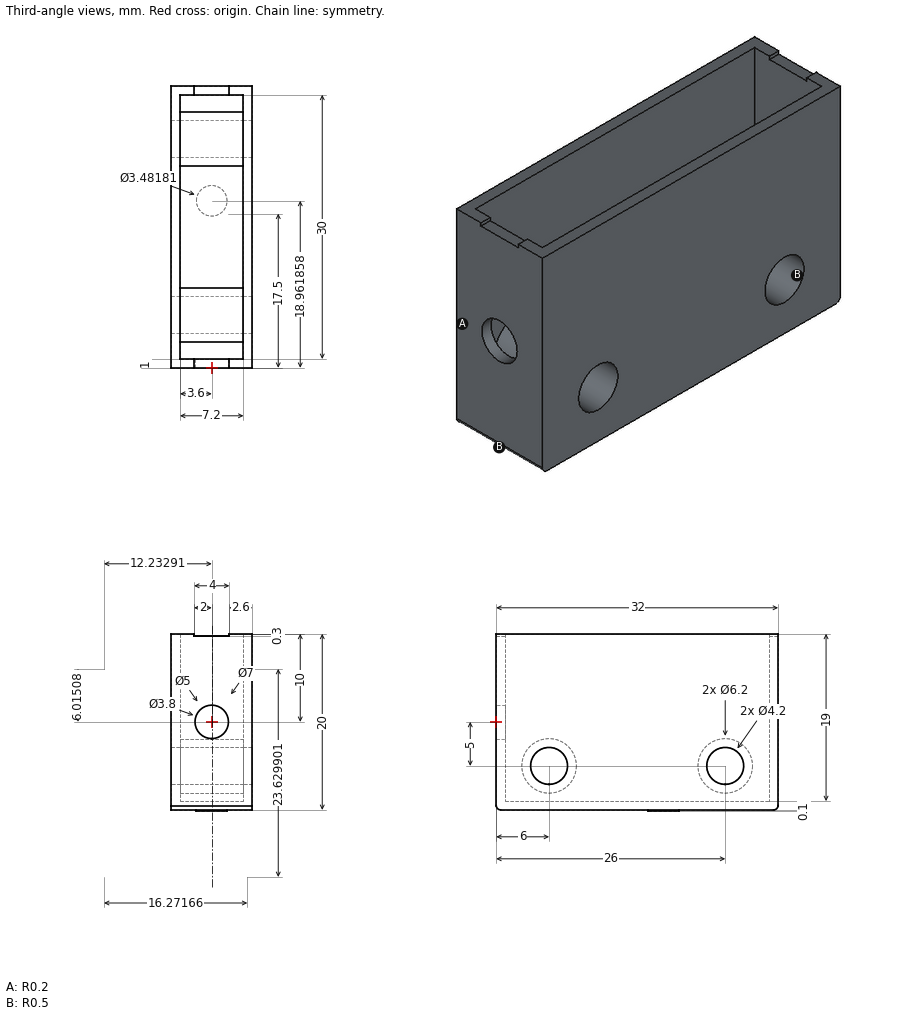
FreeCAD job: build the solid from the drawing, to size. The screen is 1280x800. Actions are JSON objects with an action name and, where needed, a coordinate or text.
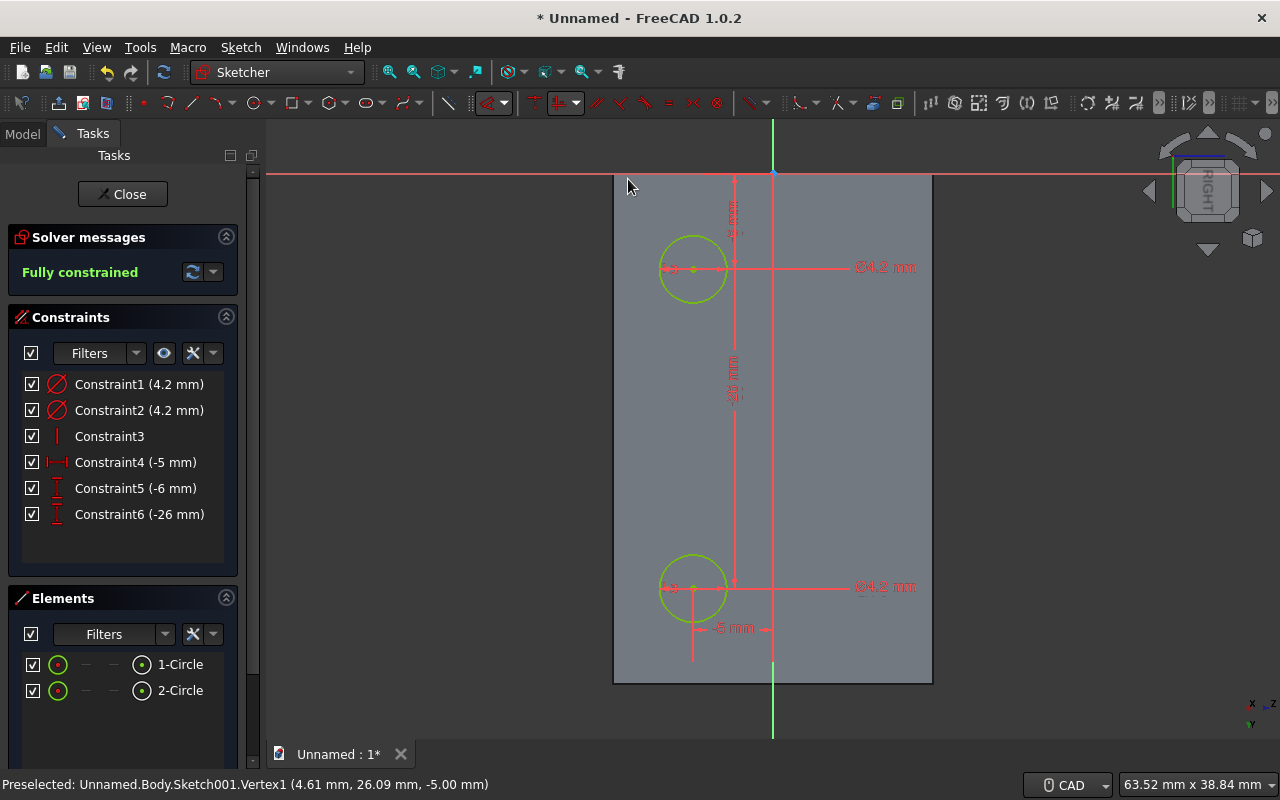
{"action": "left_click", "coordinate": [123, 194]}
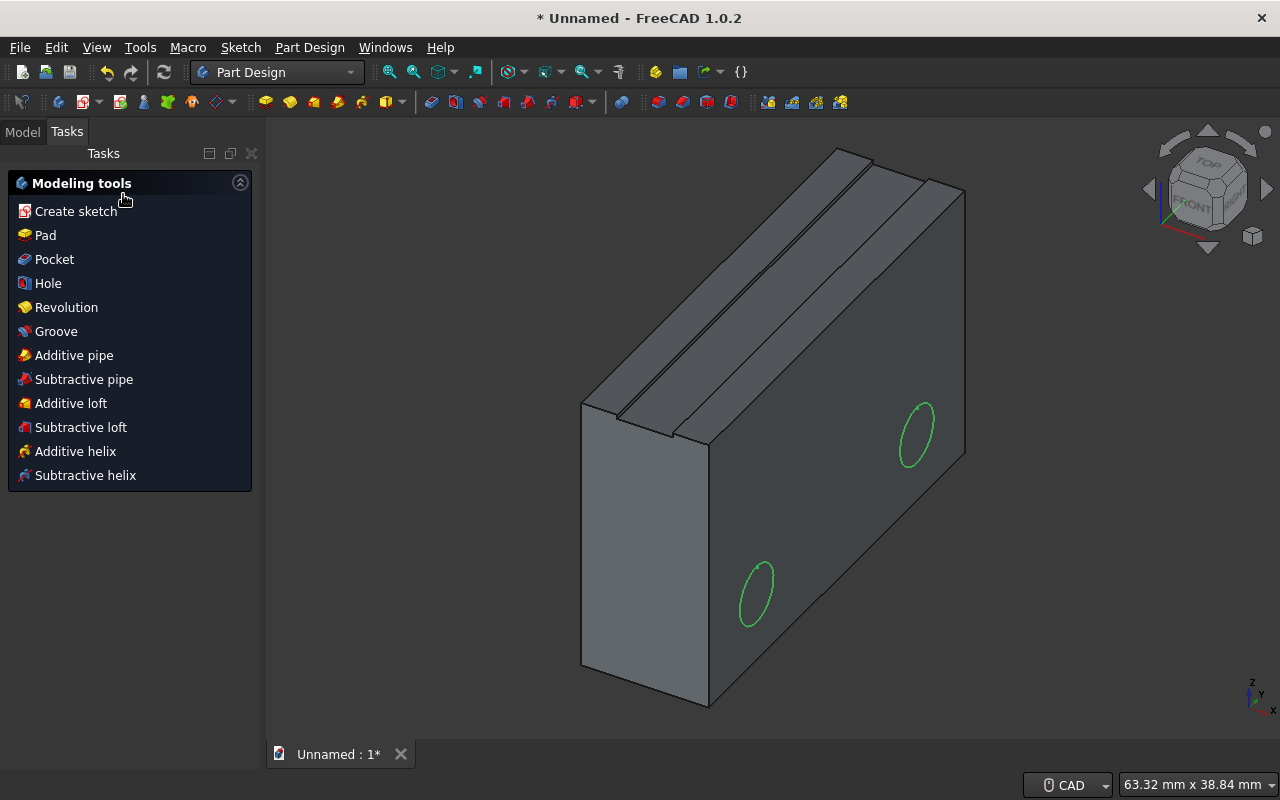
{"action": "left_click", "coordinate": [432, 102]}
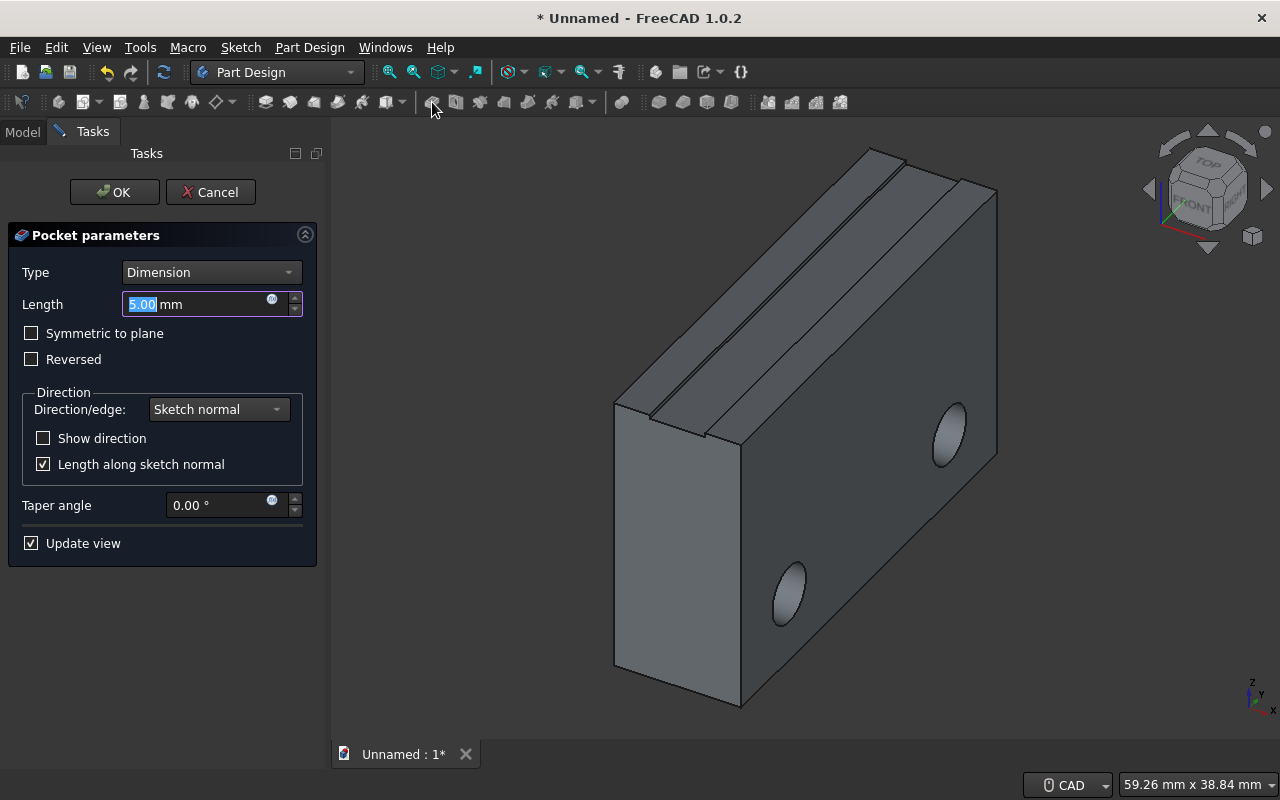
{"action": "left_click", "coordinate": [212, 272]}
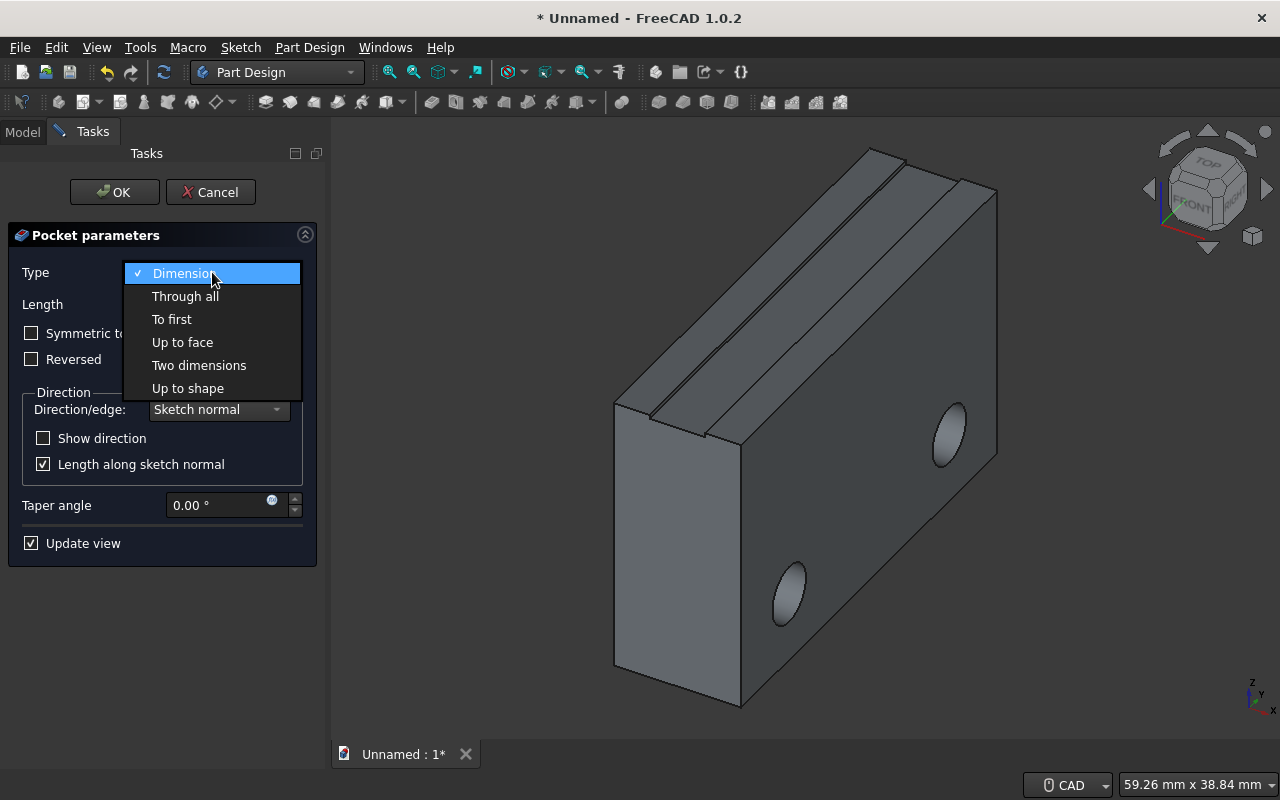
{"action": "left_click", "coordinate": [212, 296]}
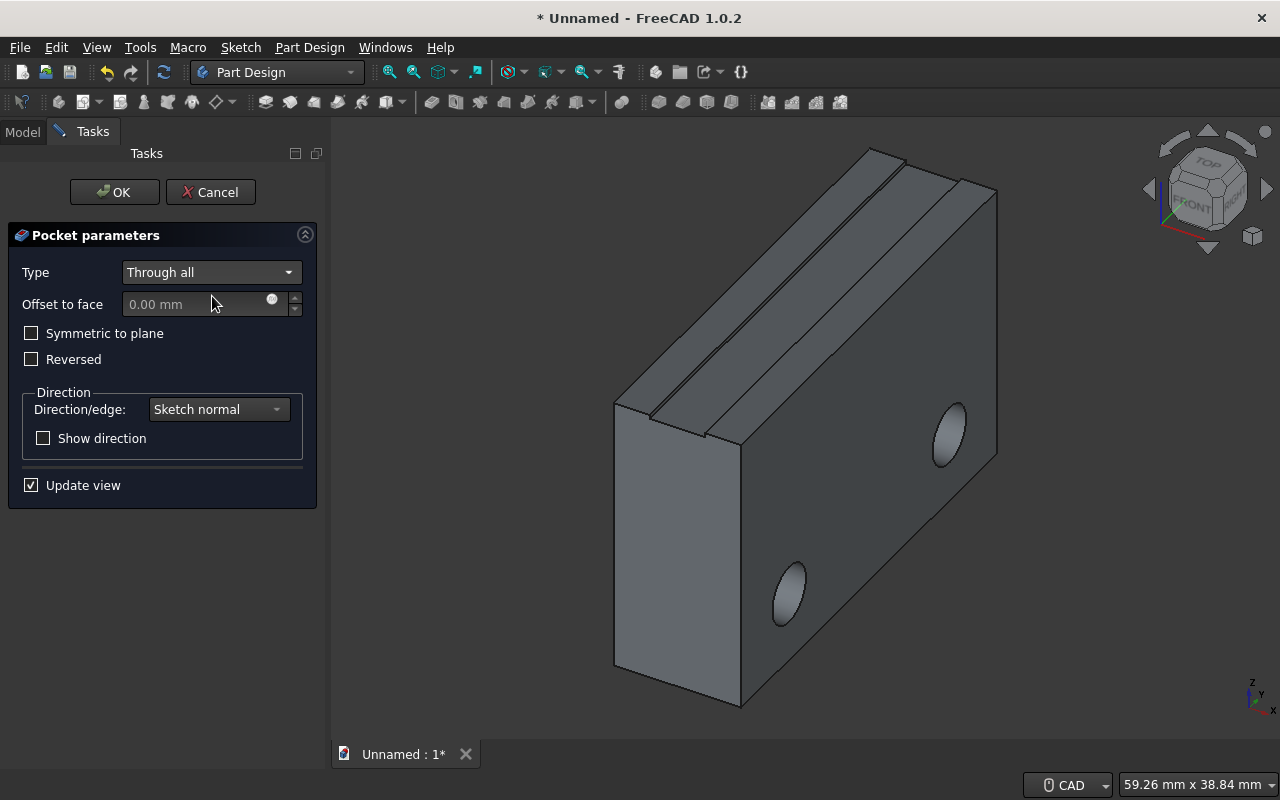
{"action": "left_click", "coordinate": [115, 192]}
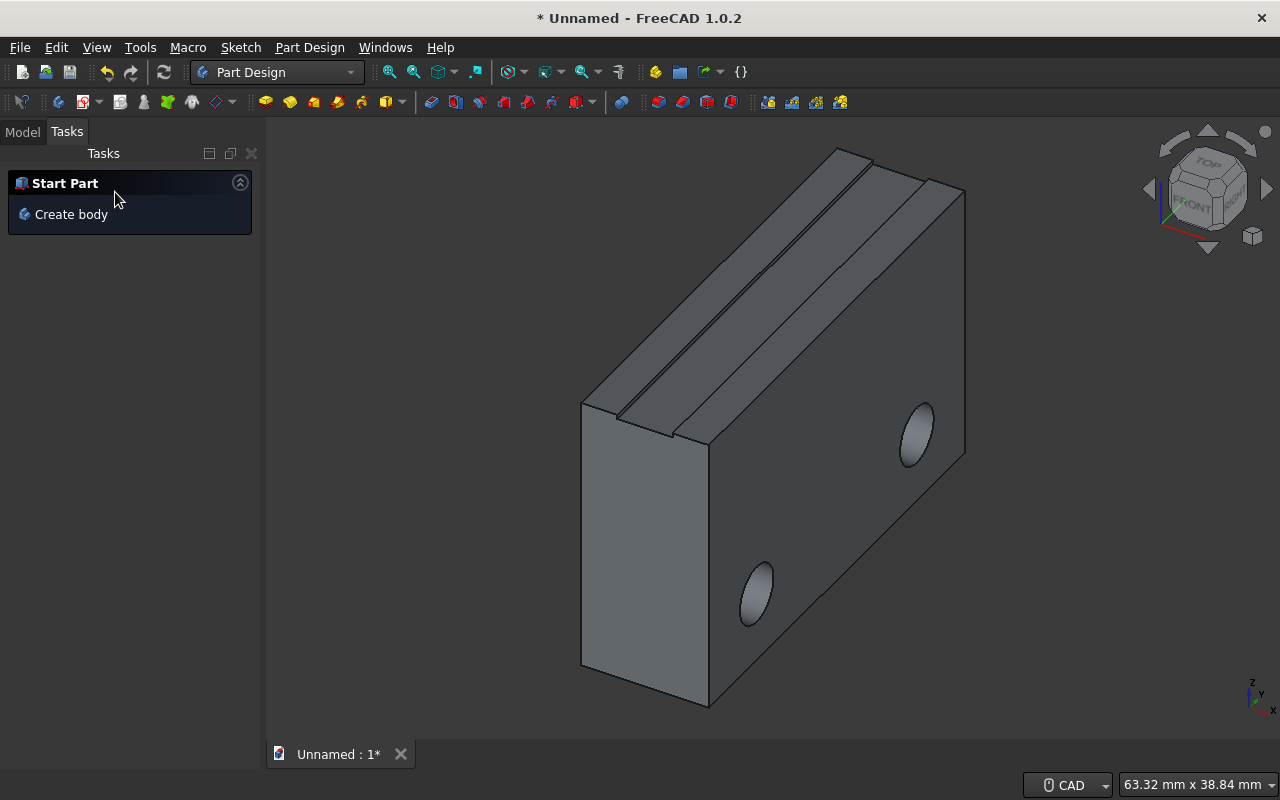
{"action": "key", "text": "5"}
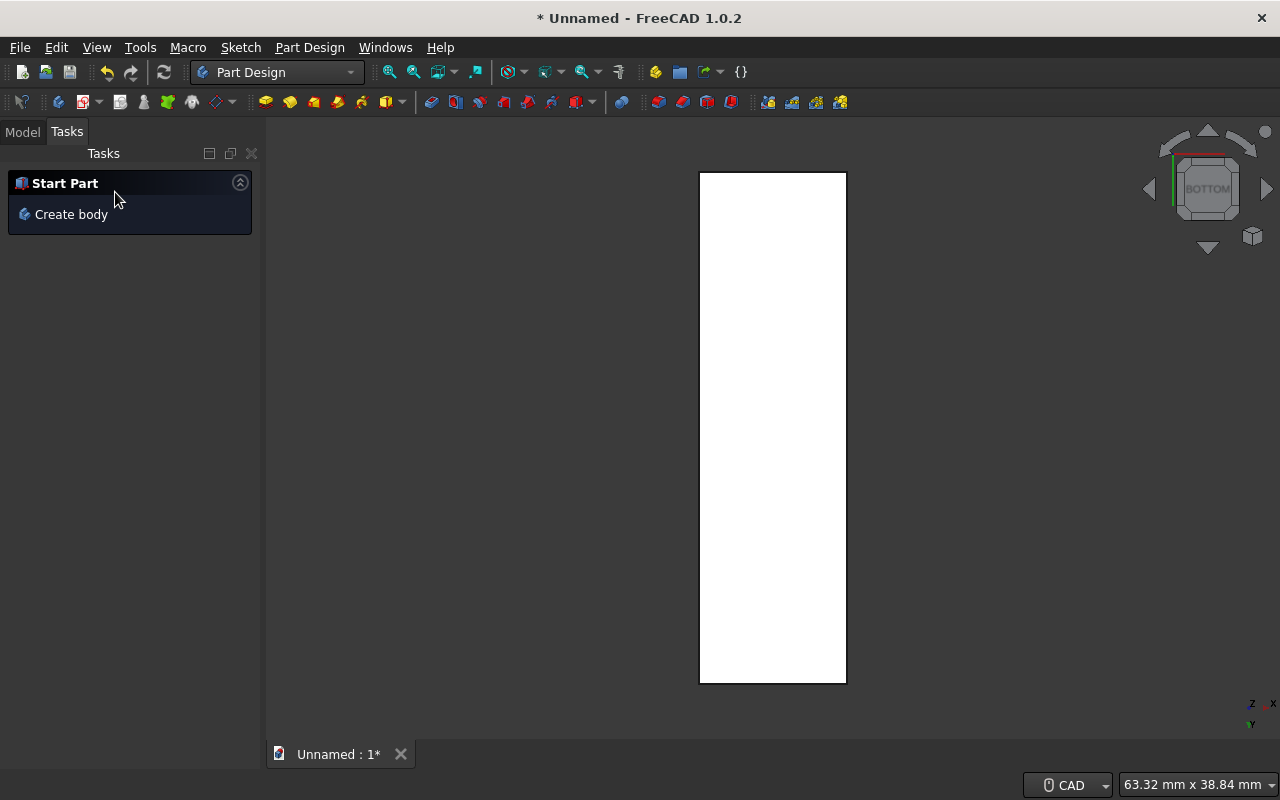
{"action": "left_click", "coordinate": [773, 573]}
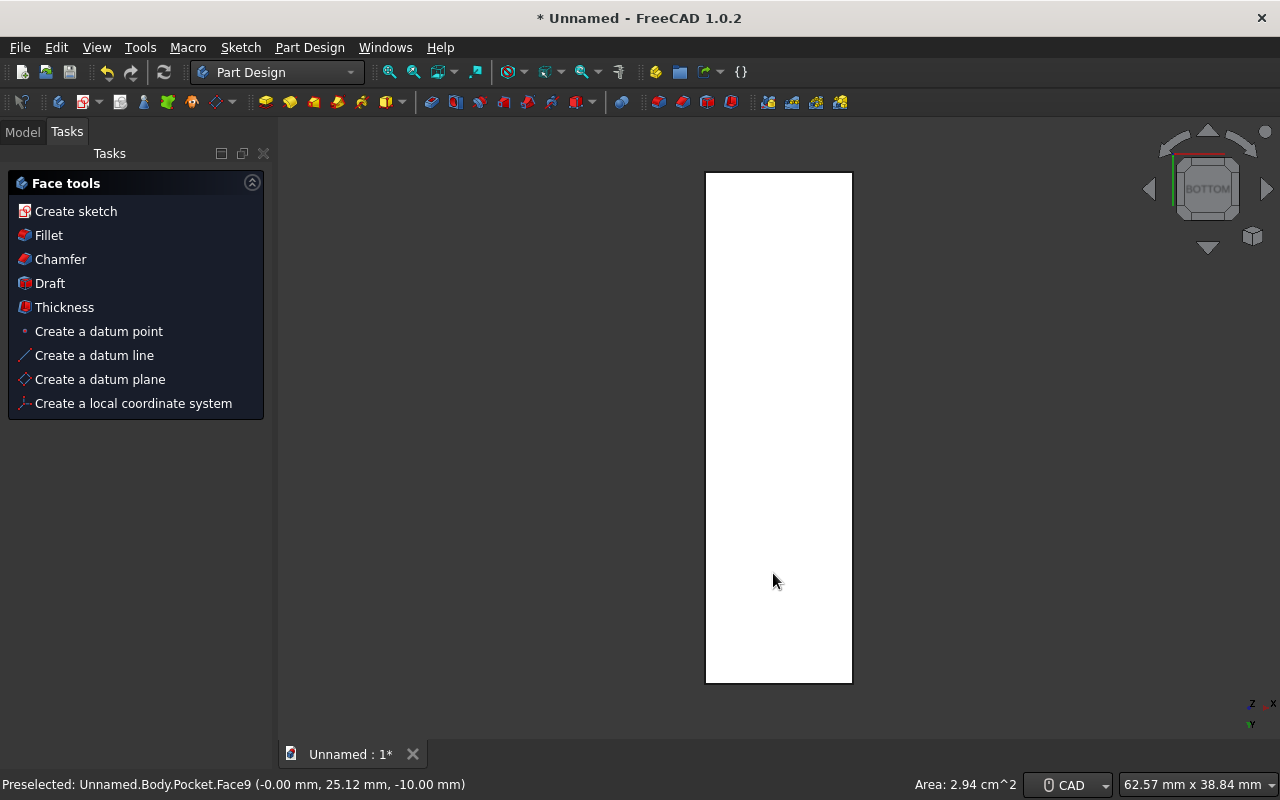
{"action": "left_click", "coordinate": [84, 102]}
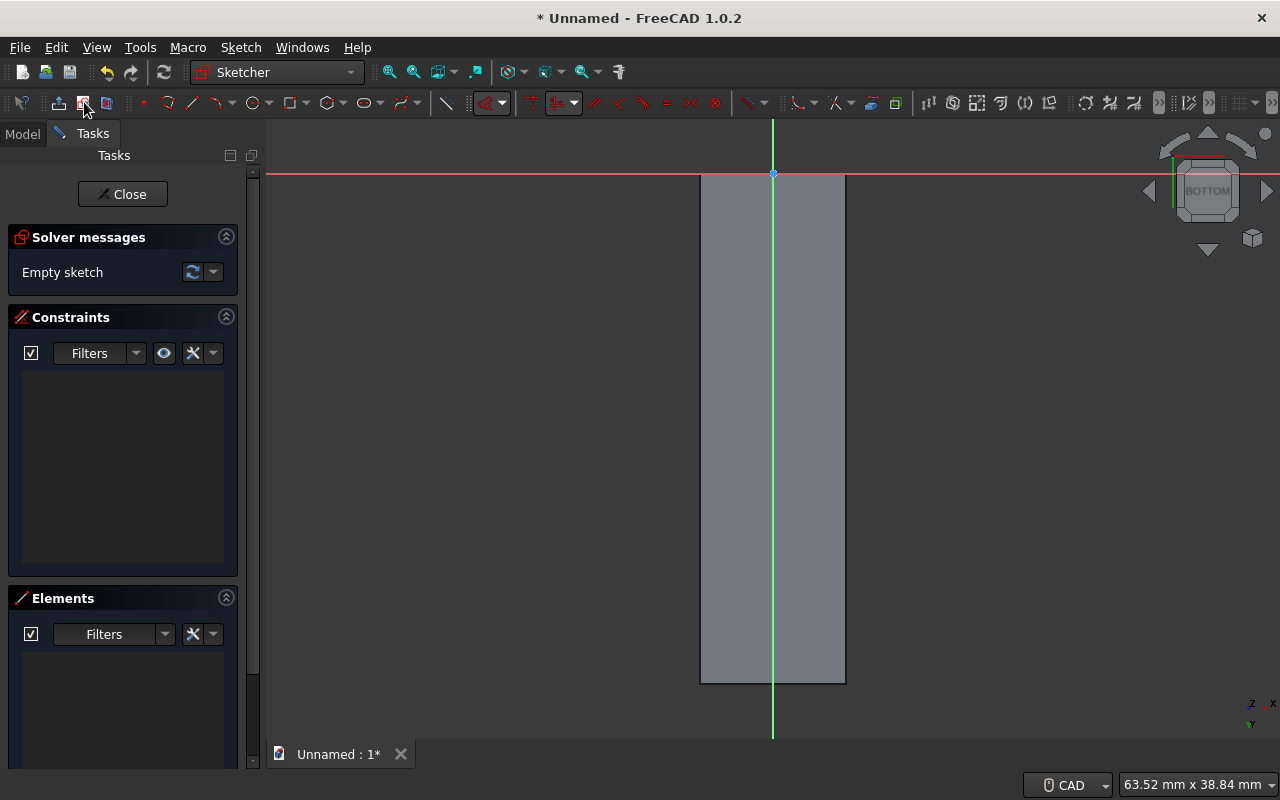
{"action": "scroll", "coordinate": [784, 484], "scroll_direction": "up", "scroll_amount": 10}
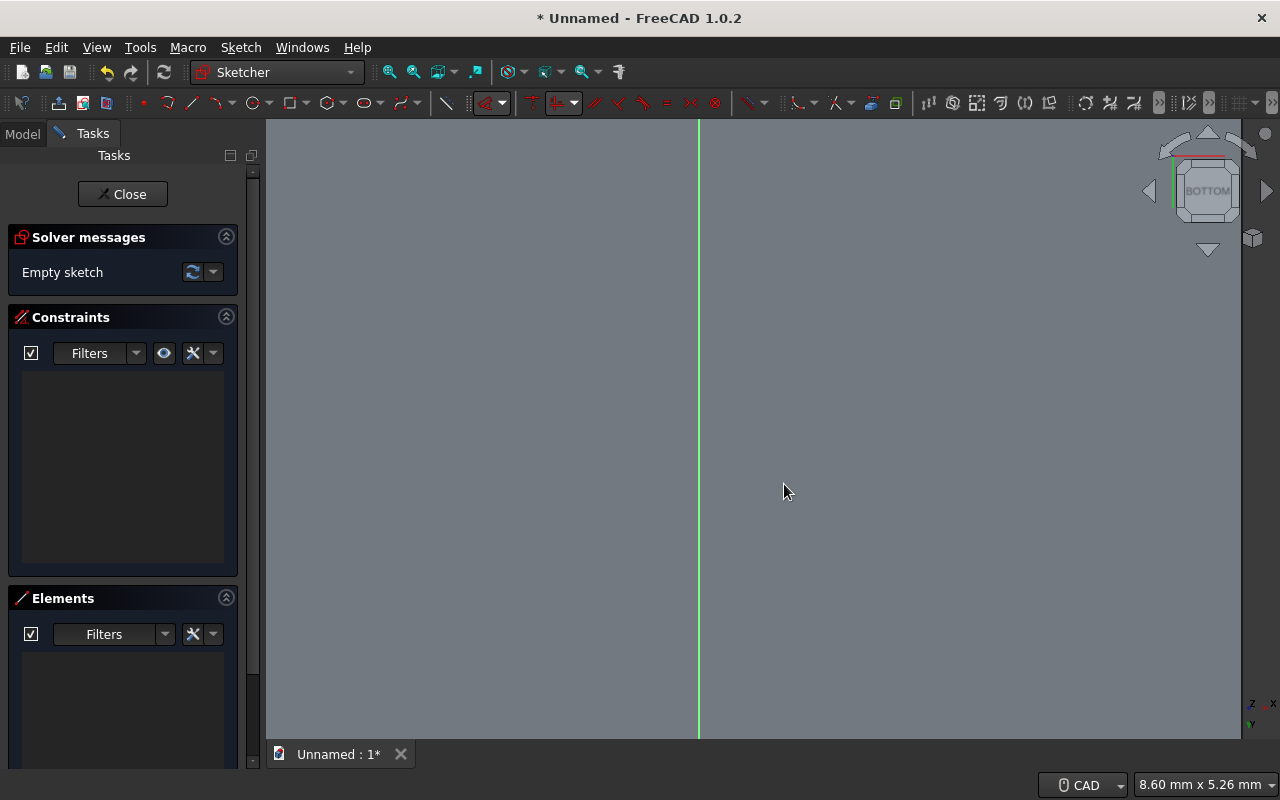
{"action": "left_click", "coordinate": [254, 104]}